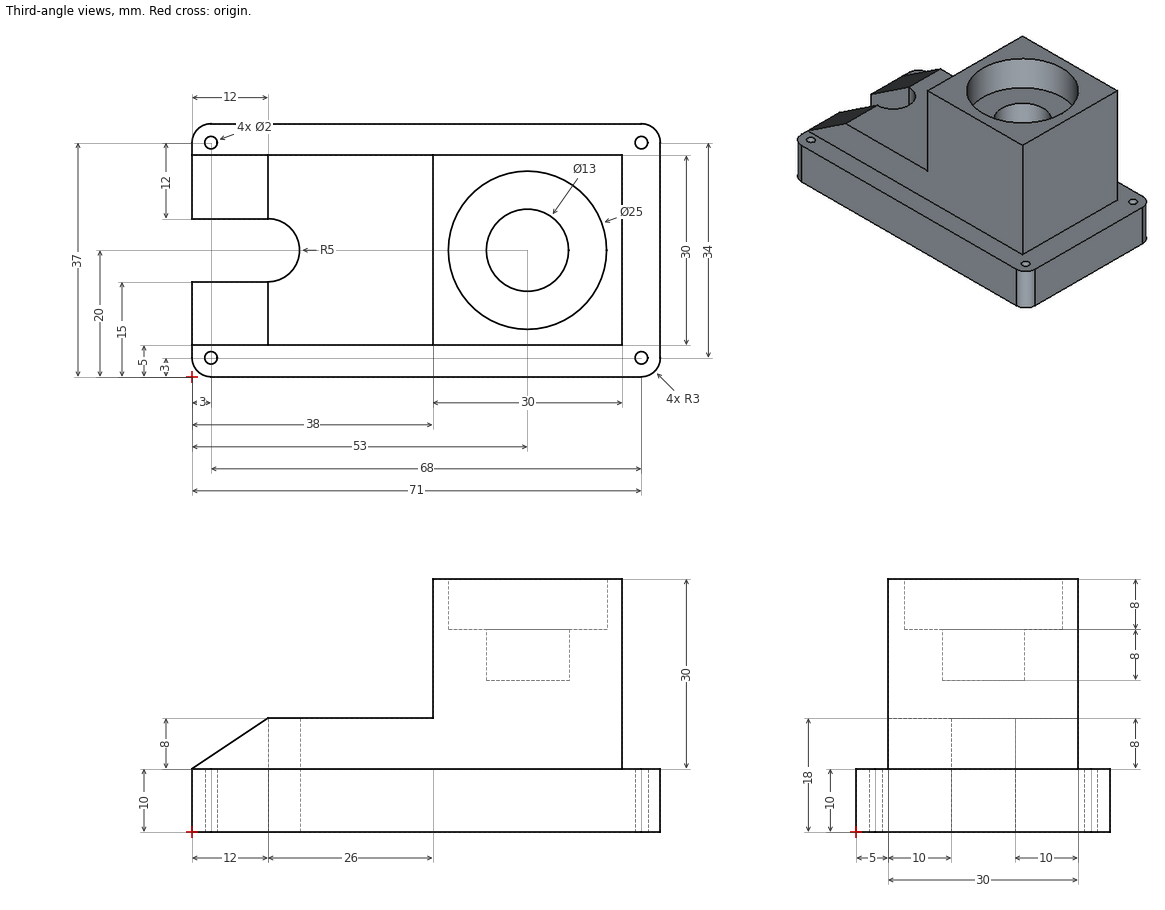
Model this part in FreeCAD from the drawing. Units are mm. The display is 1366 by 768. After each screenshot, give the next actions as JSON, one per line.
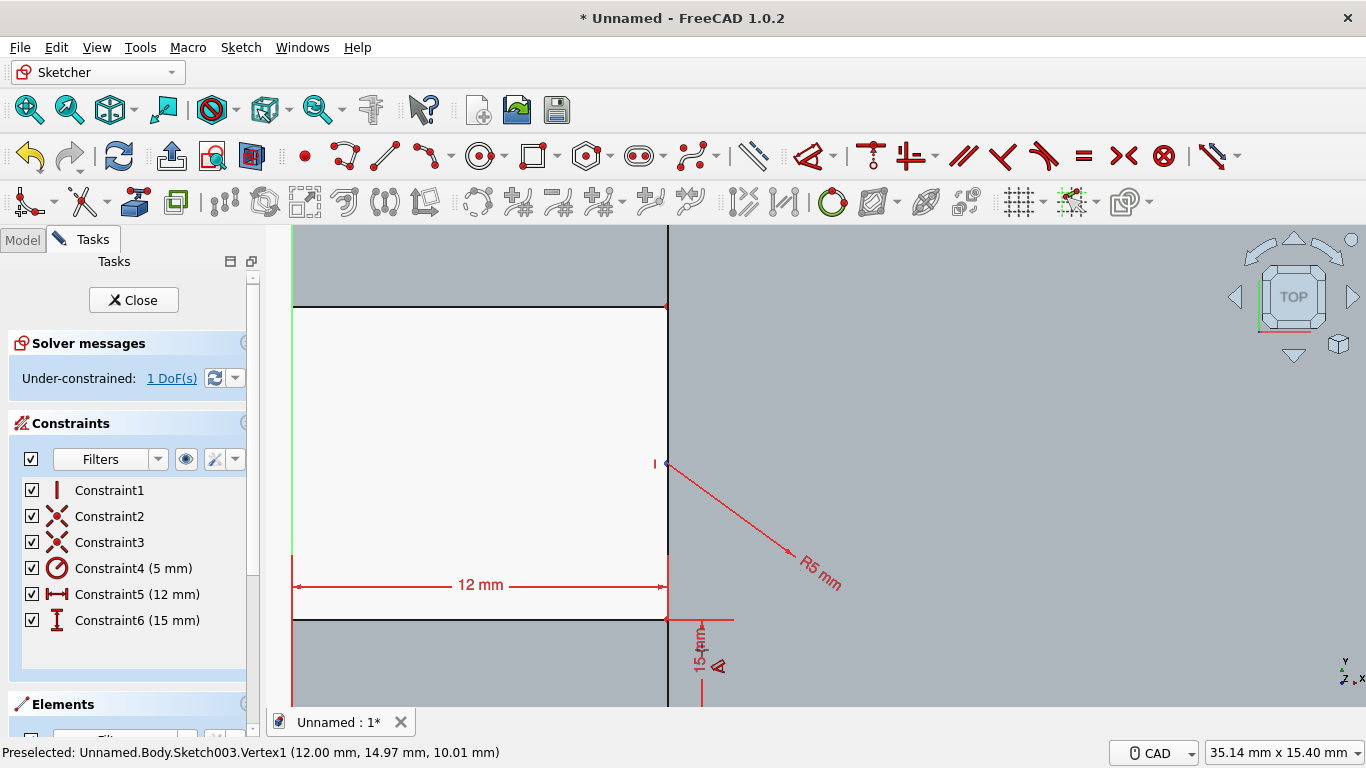
{"action": "left_click", "coordinate": [668, 463]}
{"action": "left_click", "coordinate": [481, 429]}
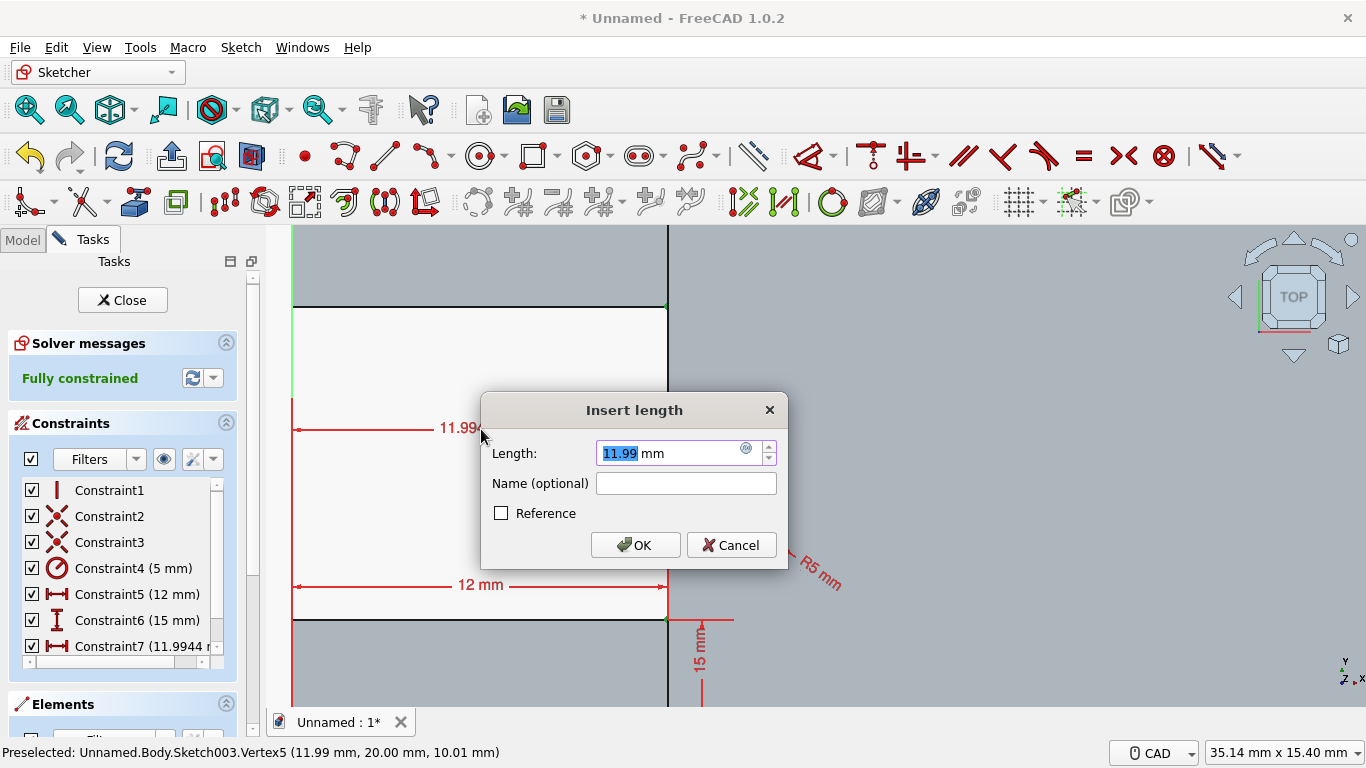
{"action": "type", "text": "12"}
{"action": "key", "text": "Return"}
{"action": "key", "text": "Escape"}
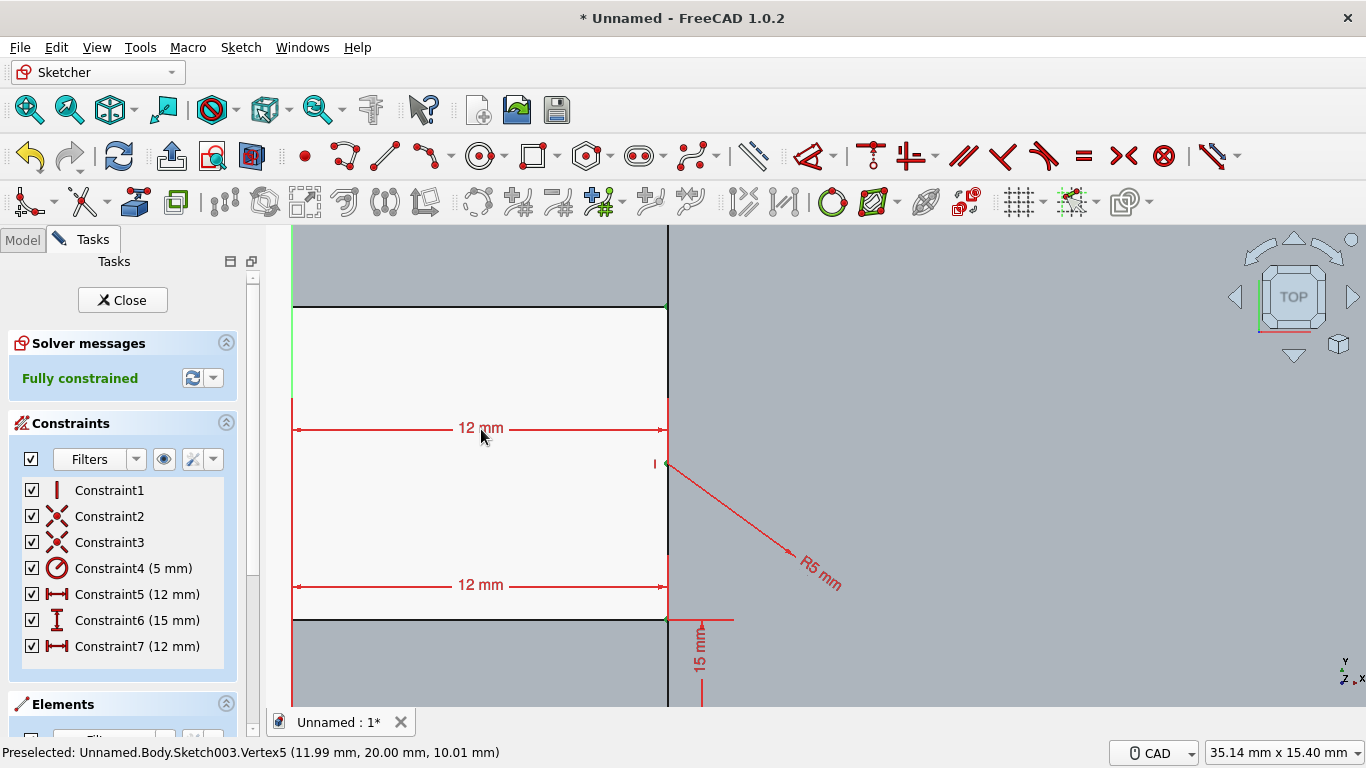
{"action": "left_click", "coordinate": [123, 300]}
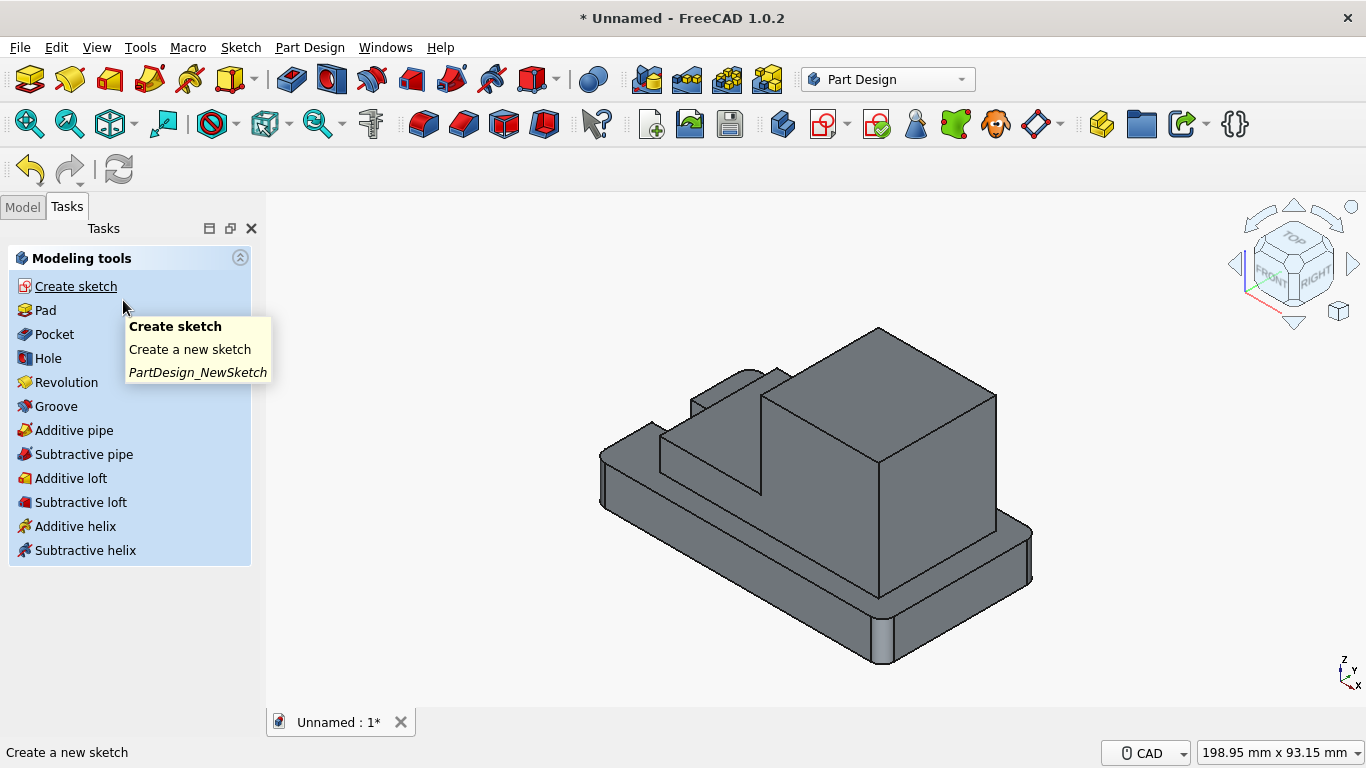
{"action": "left_click", "coordinate": [292, 80]}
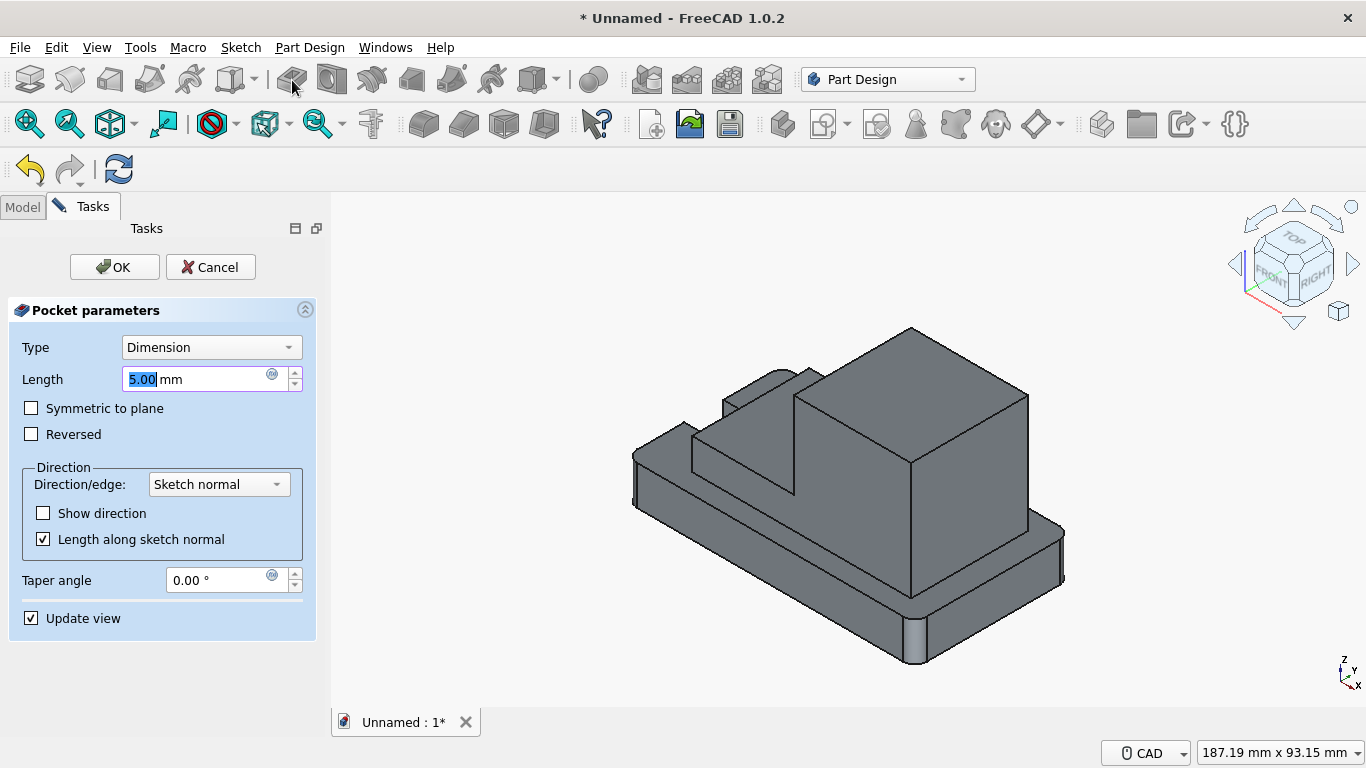
{"action": "type", "text": "8"}
{"action": "key", "text": "Tab"}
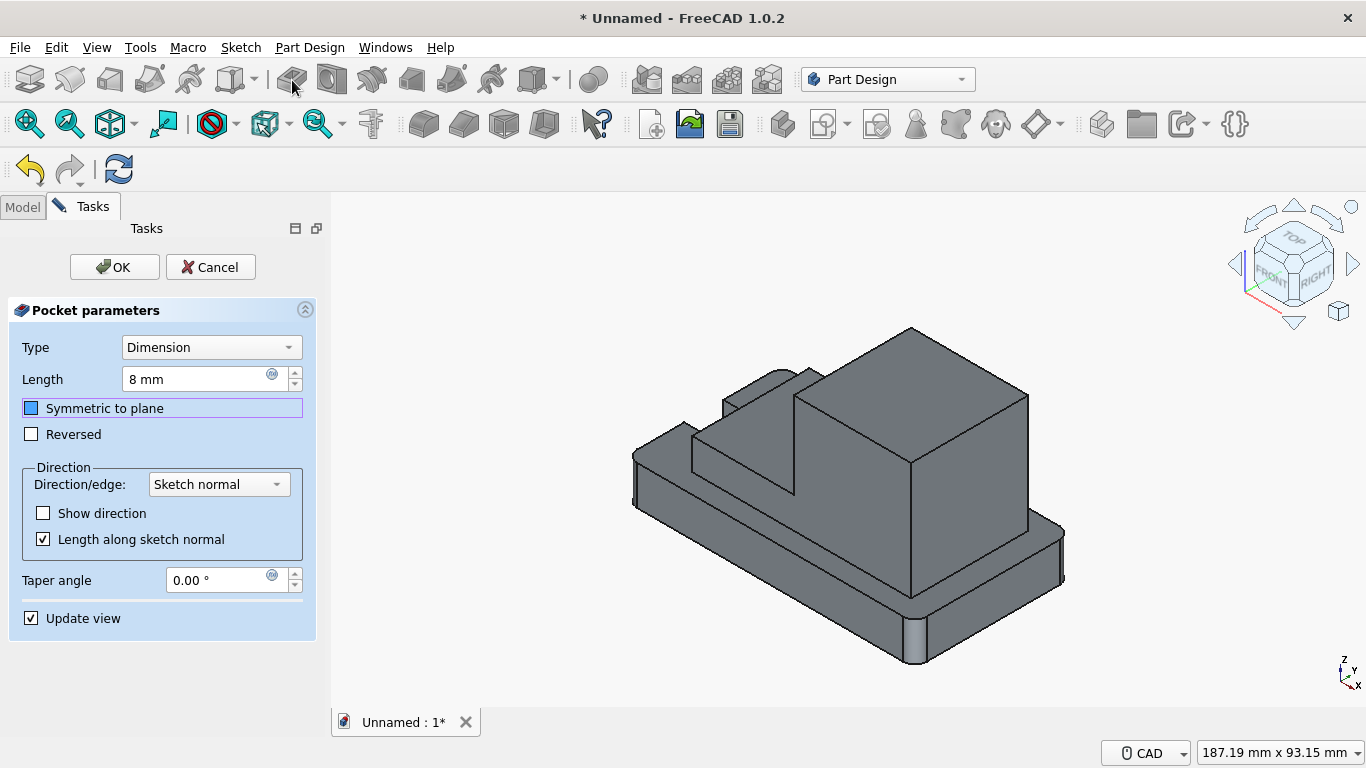
{"action": "left_click", "coordinate": [30, 434]}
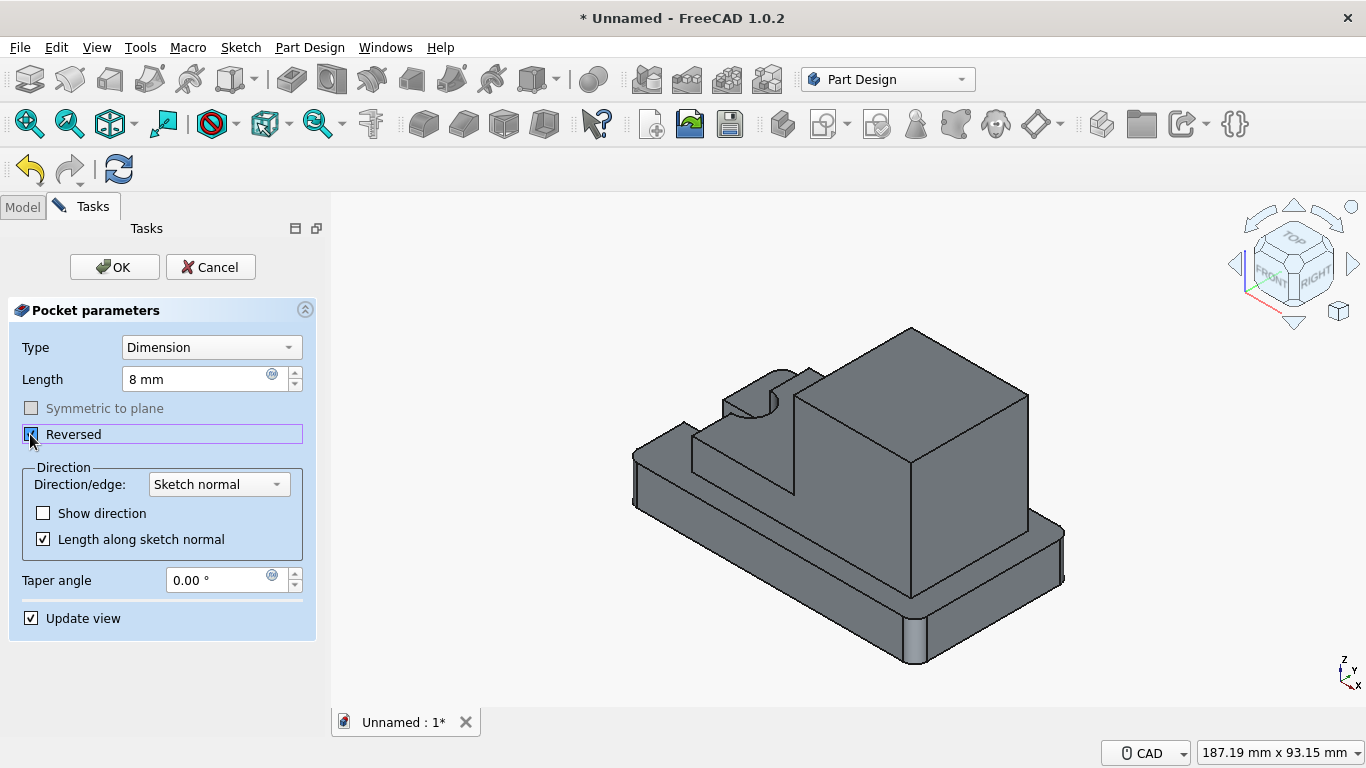
{"action": "left_click", "coordinate": [115, 267]}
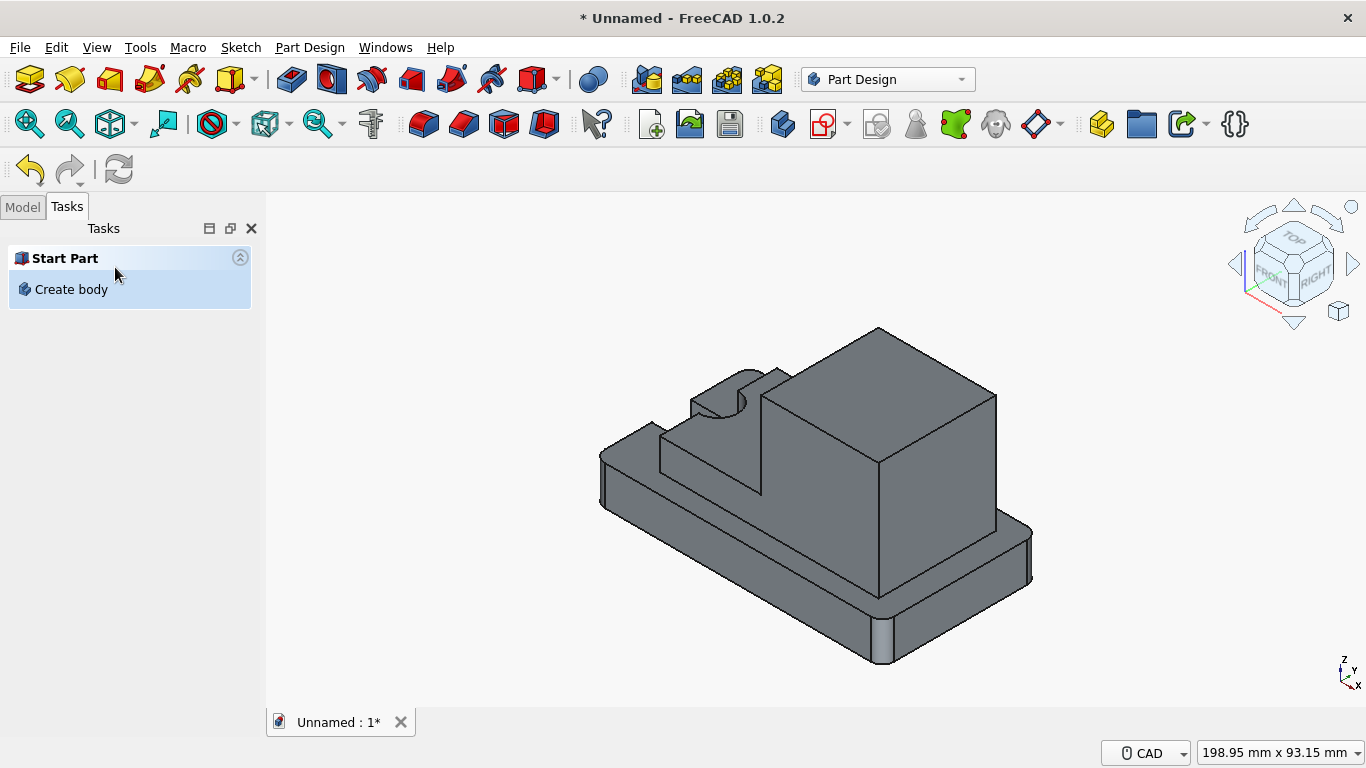
{"action": "left_click", "coordinate": [832, 503]}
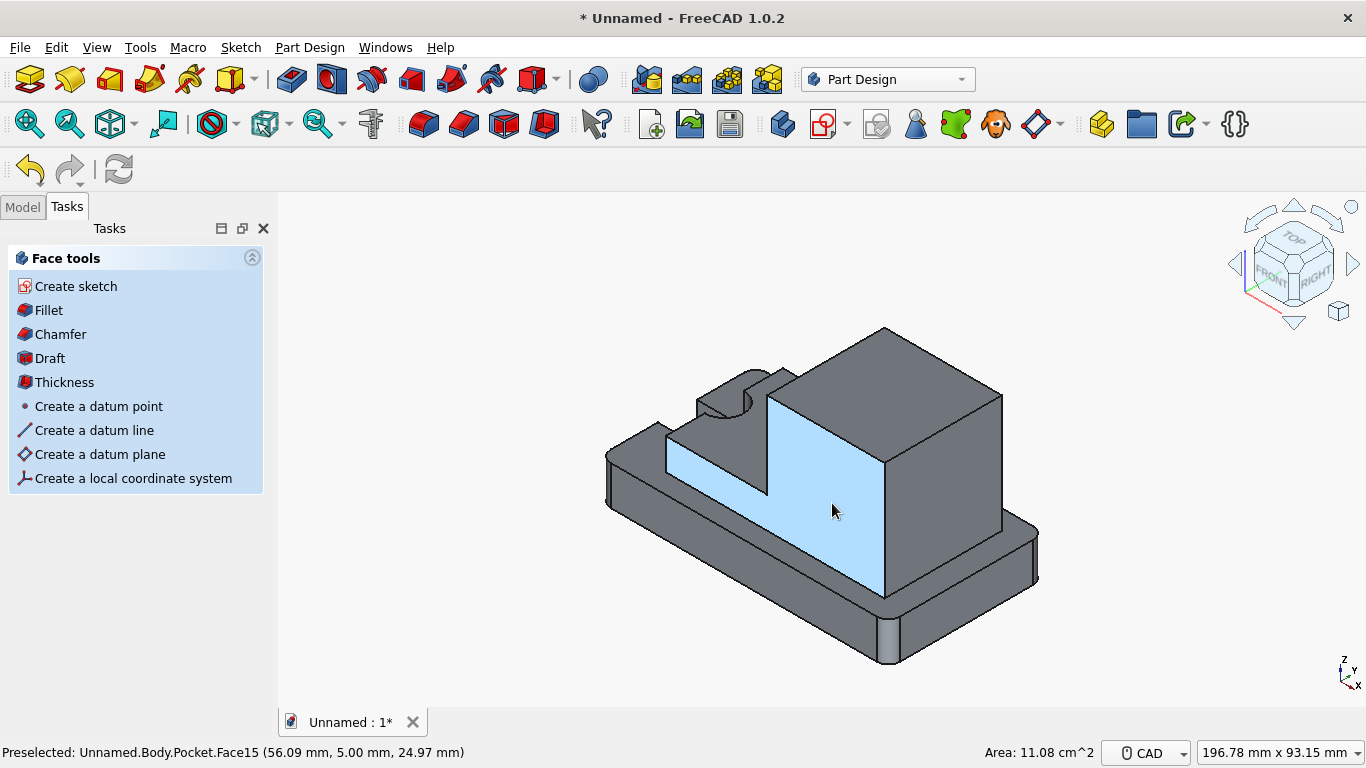
{"action": "left_click", "coordinate": [824, 124]}